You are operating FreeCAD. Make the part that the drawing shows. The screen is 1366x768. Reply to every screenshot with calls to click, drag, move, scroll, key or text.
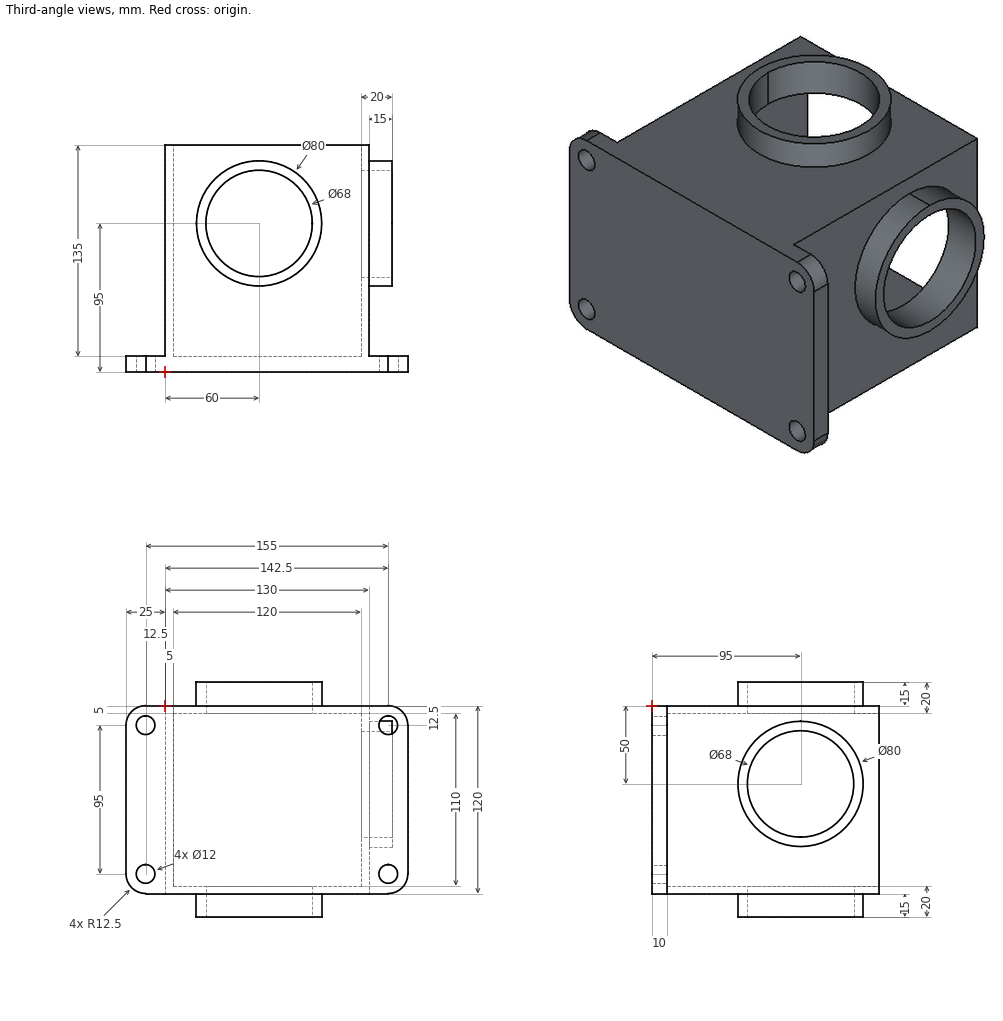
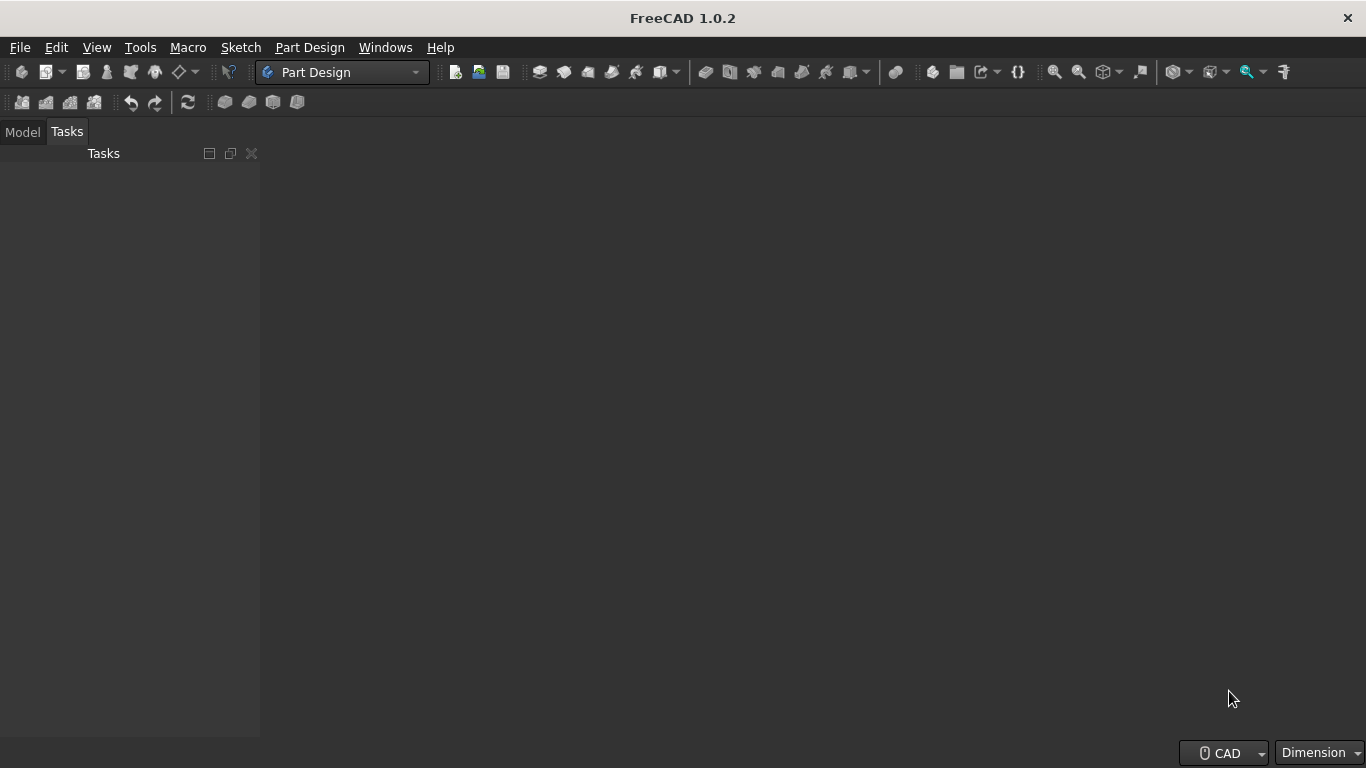
key(ctrl+n)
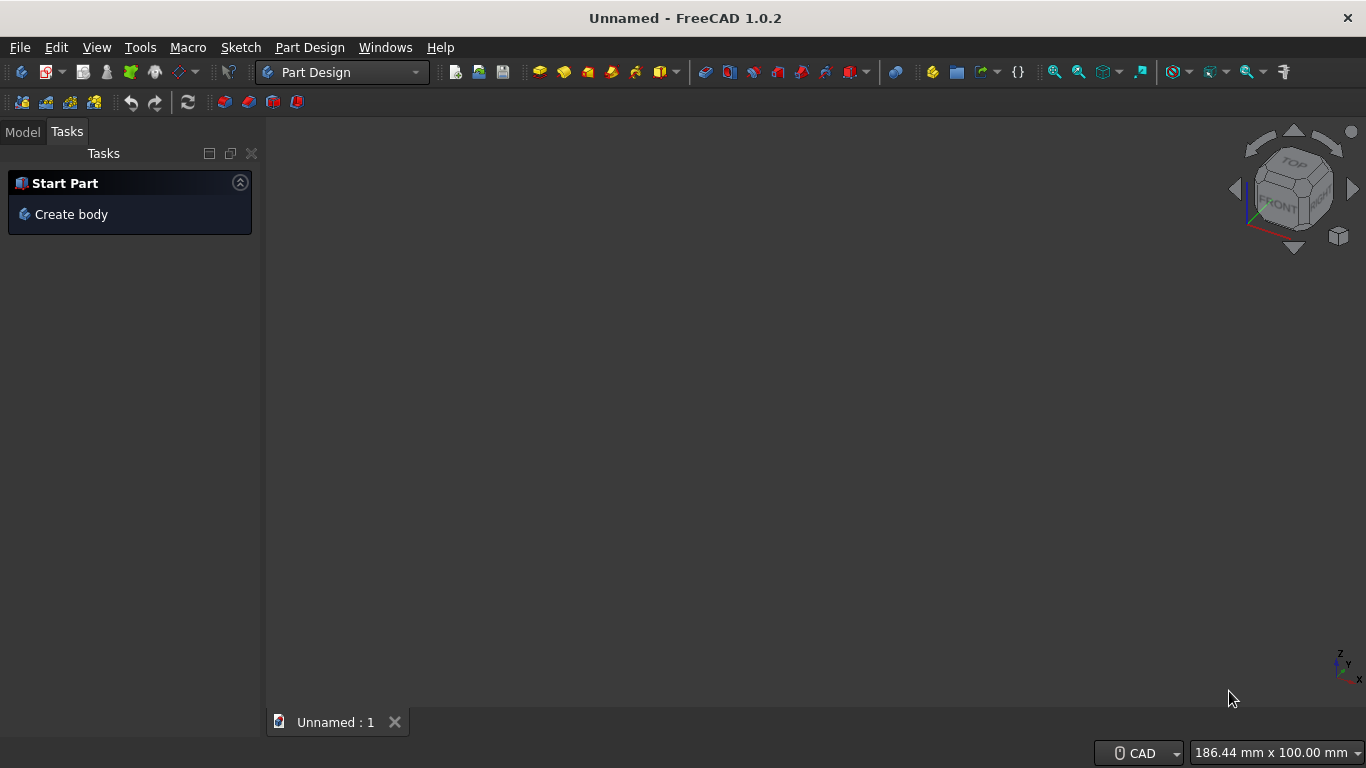
click(46, 72)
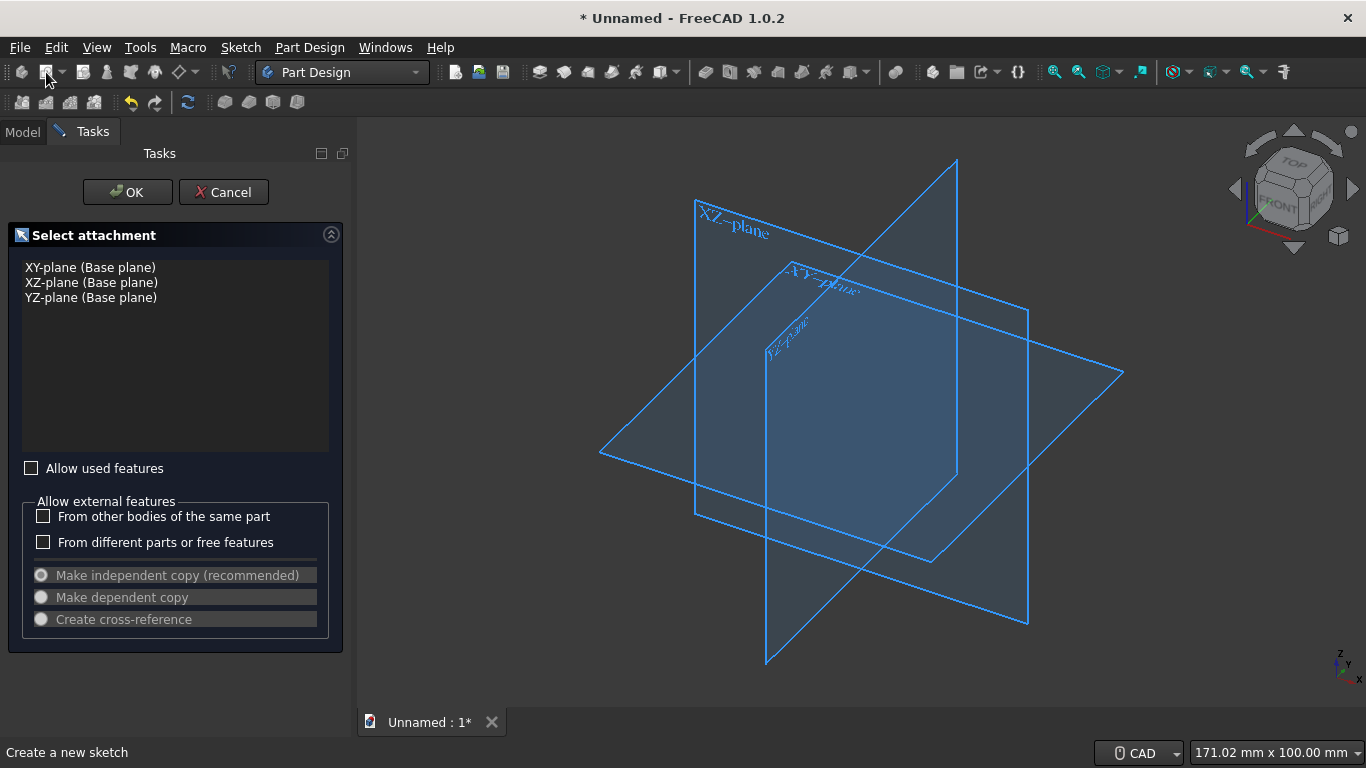
click(82, 282)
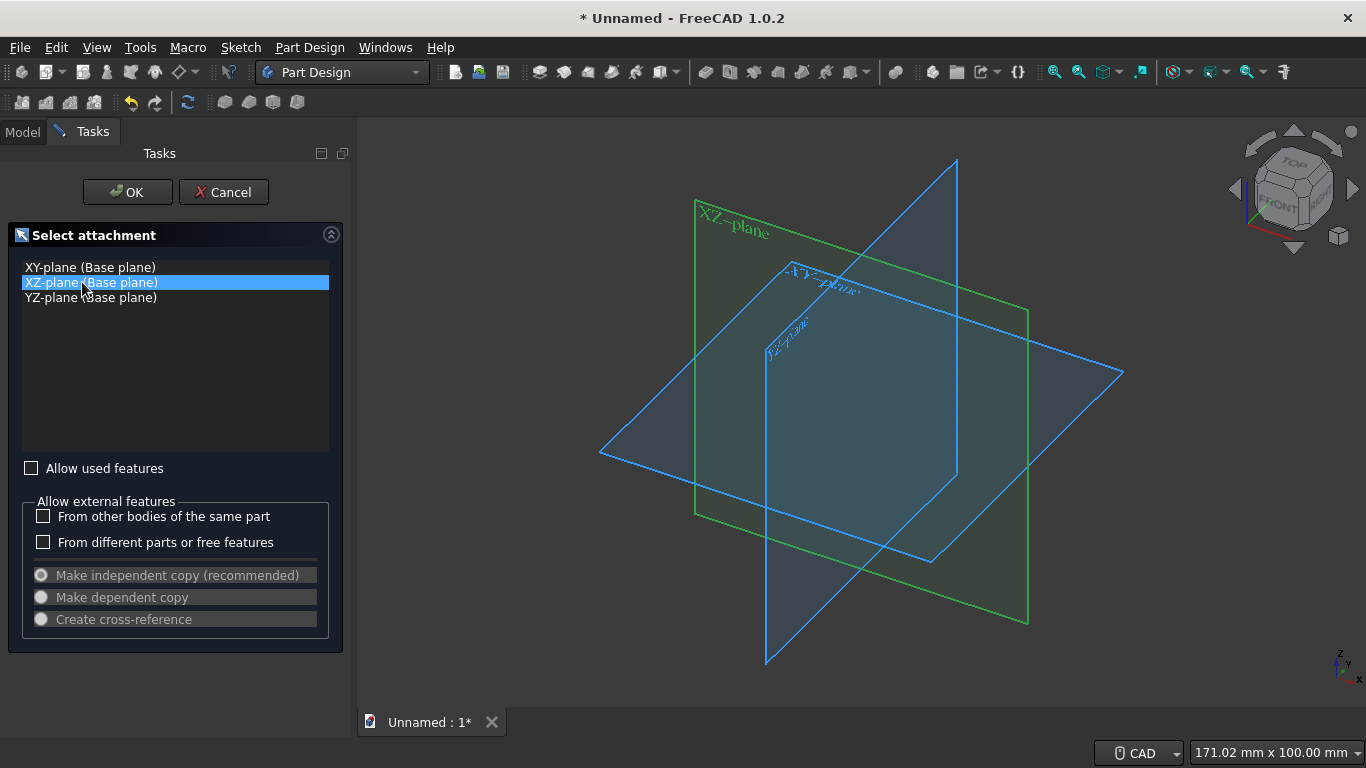
click(128, 192)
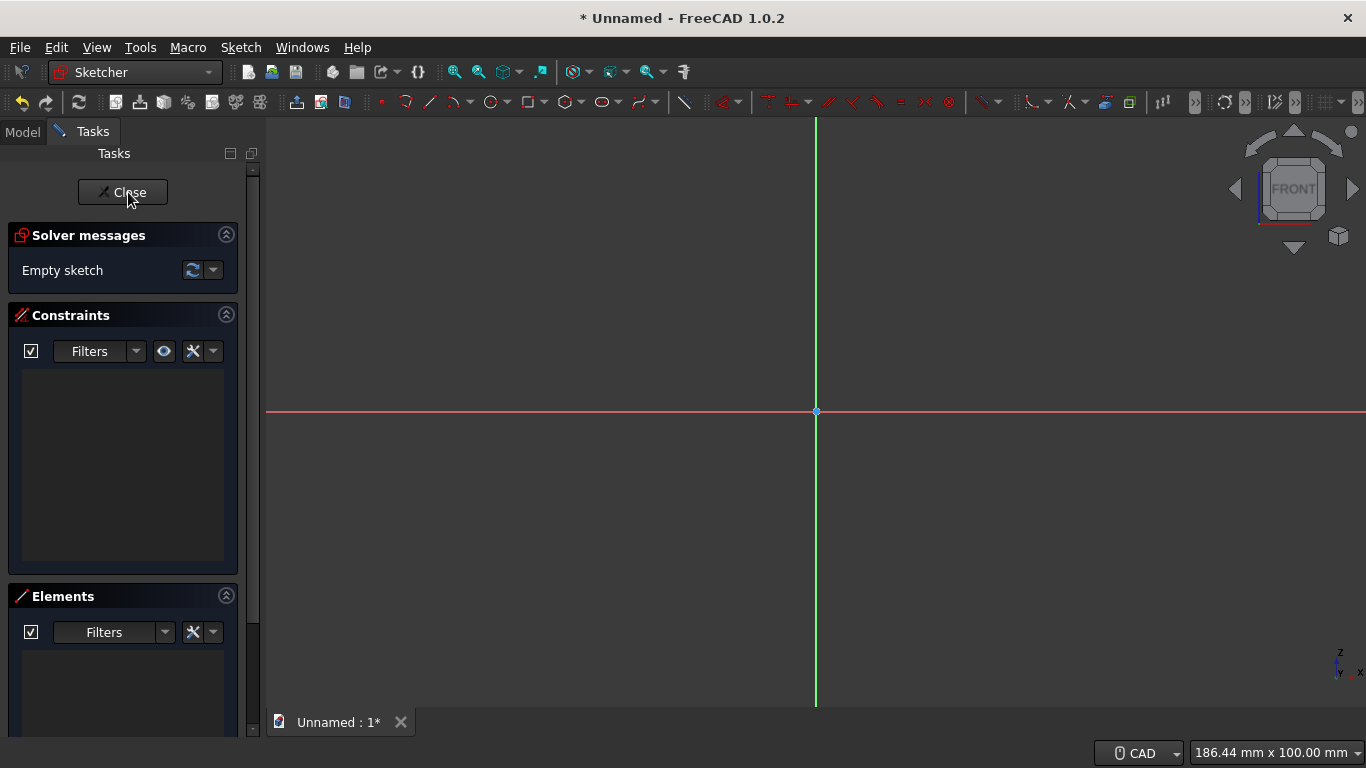
scroll(379, 145, down, 4)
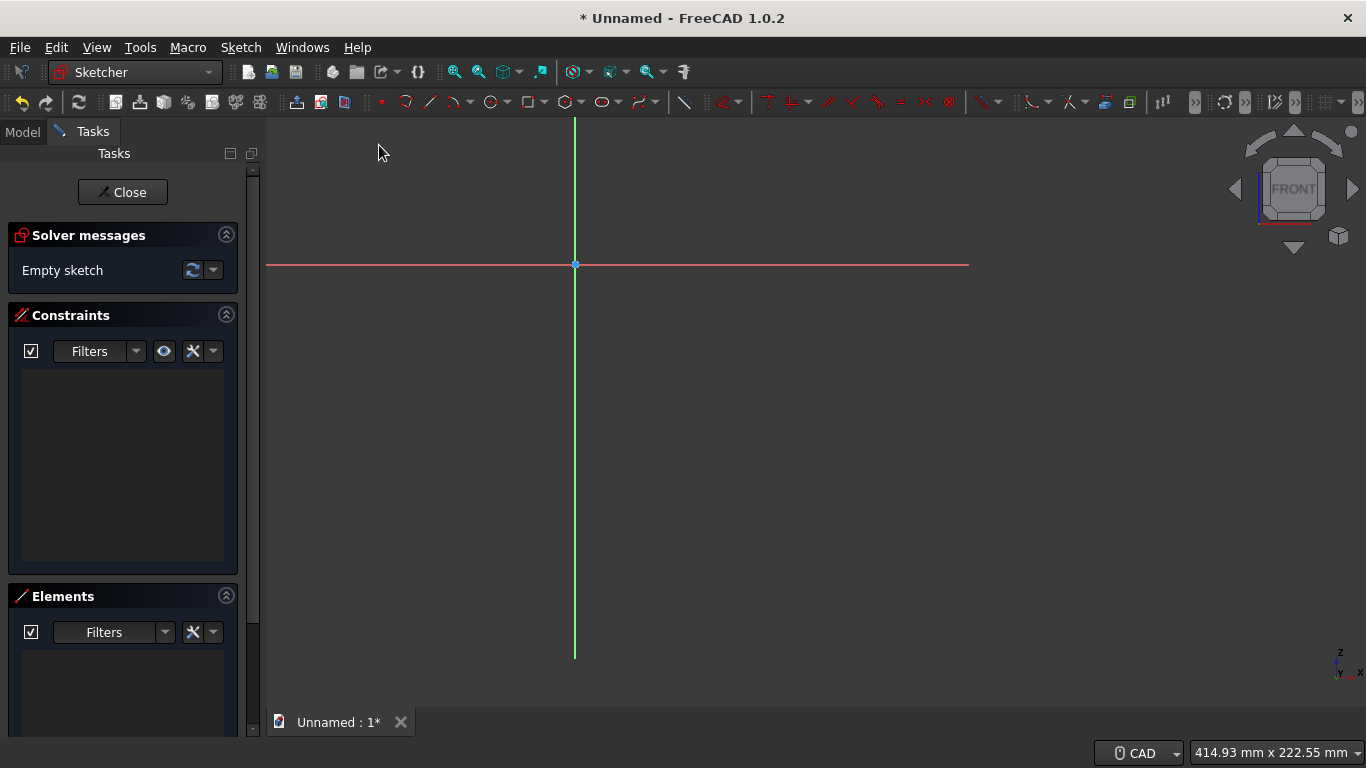
click(430, 102)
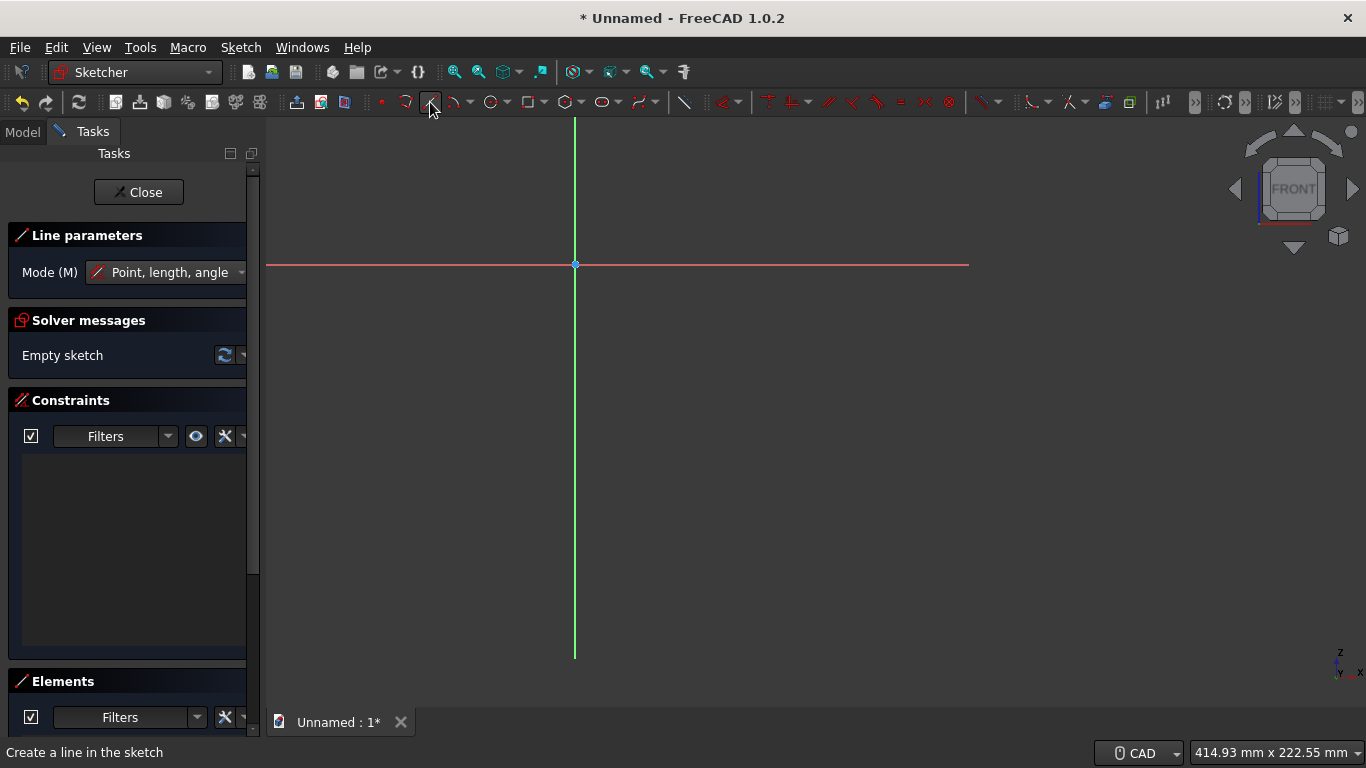
click(509, 550)
click(509, 298)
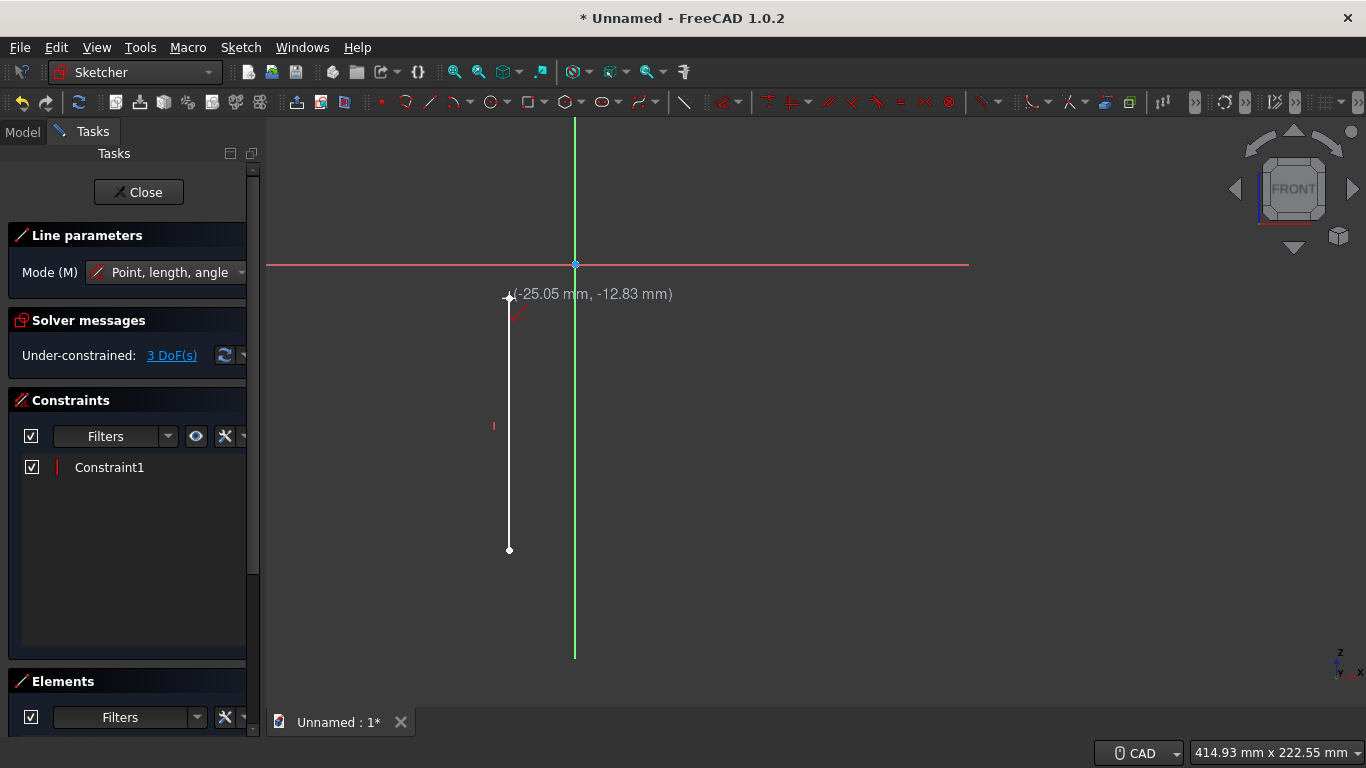
click(542, 265)
click(953, 274)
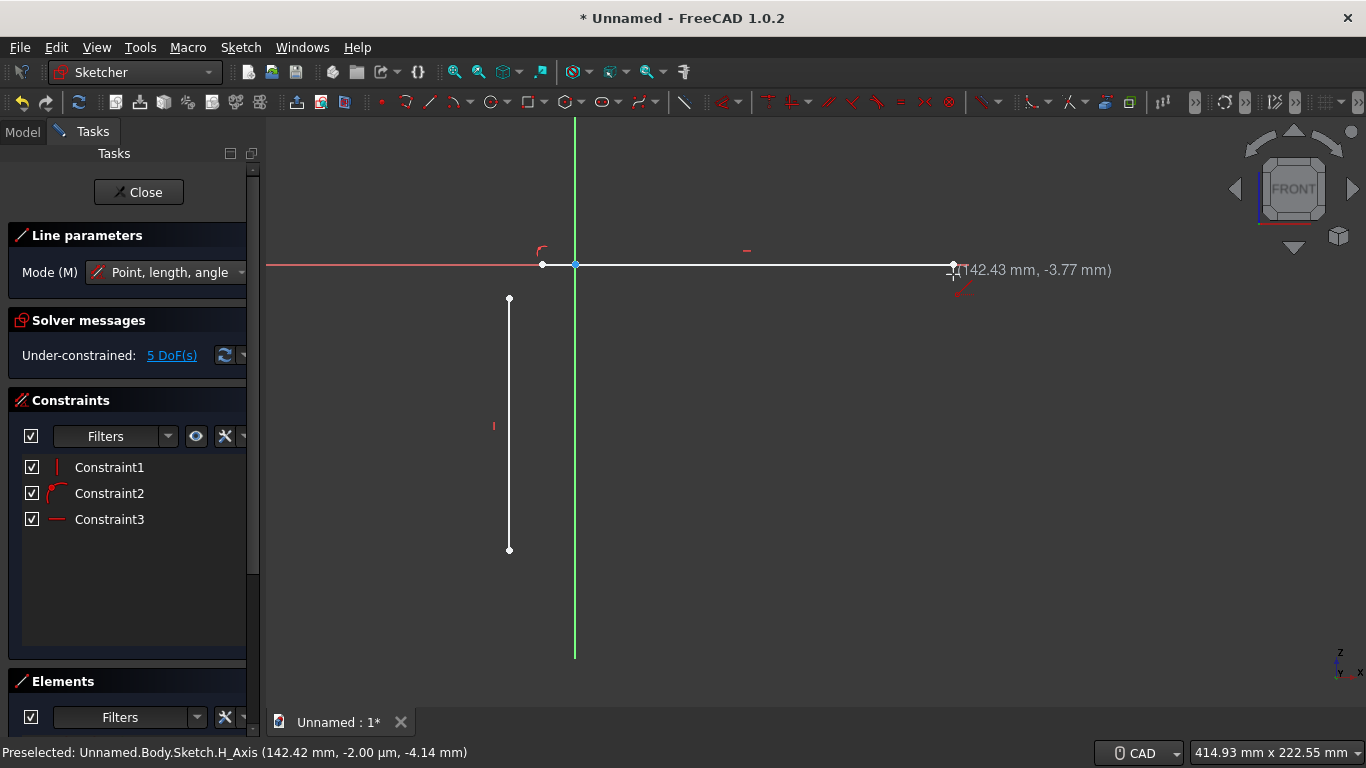
click(986, 298)
click(986, 550)